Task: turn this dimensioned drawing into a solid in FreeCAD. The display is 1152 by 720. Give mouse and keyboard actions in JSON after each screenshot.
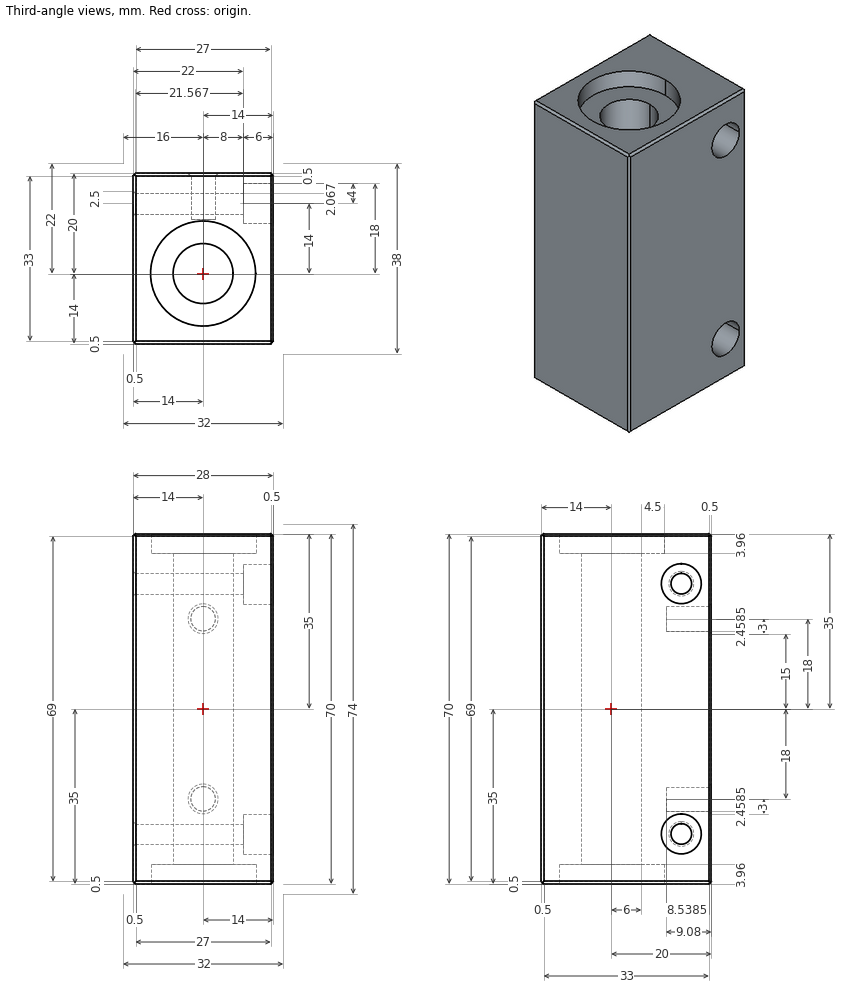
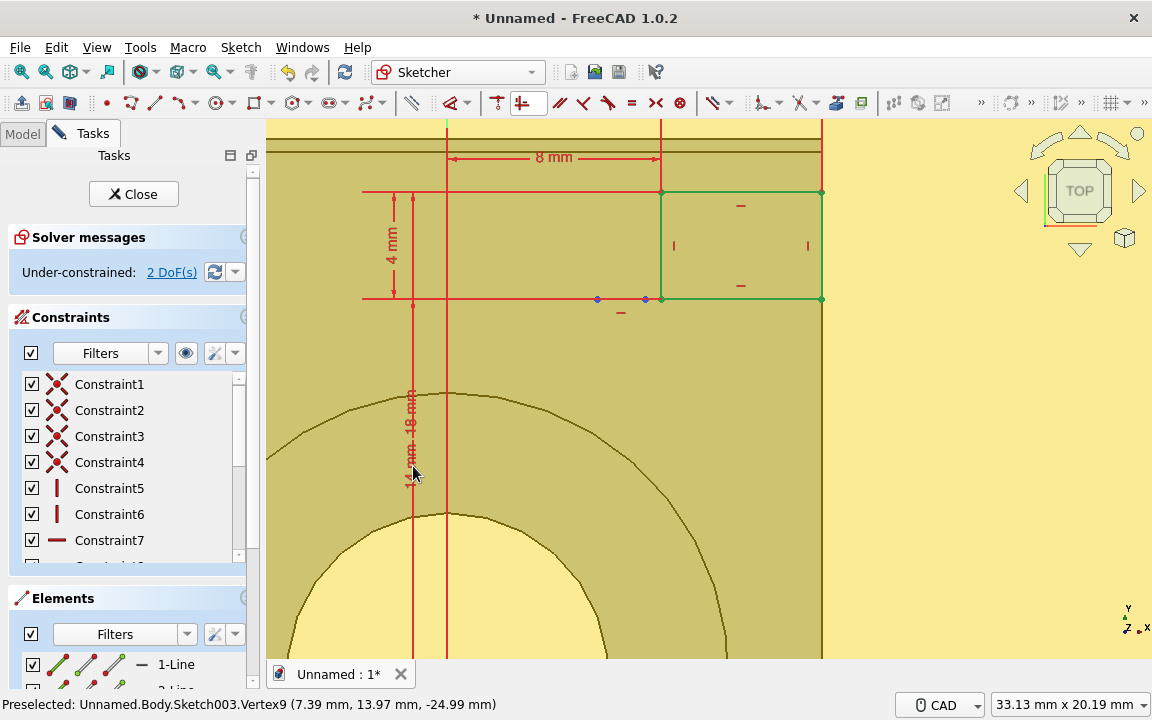
{"action": "left_click", "coordinate": [134, 194]}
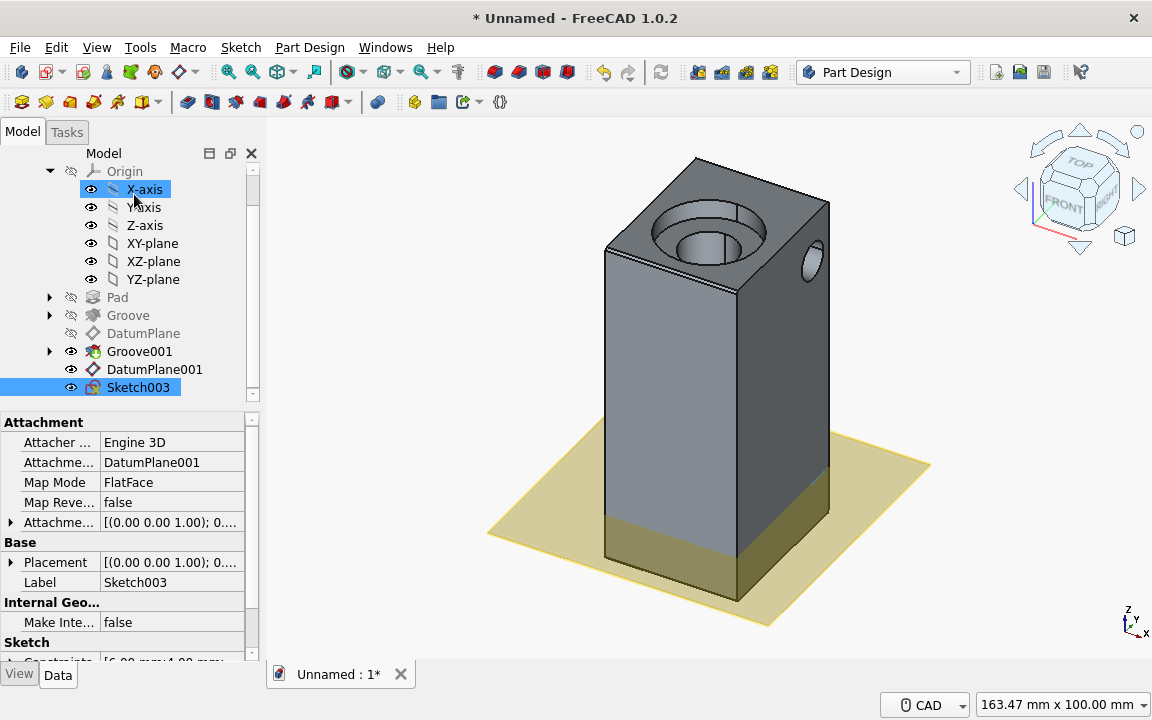
{"action": "left_click", "coordinate": [236, 102]}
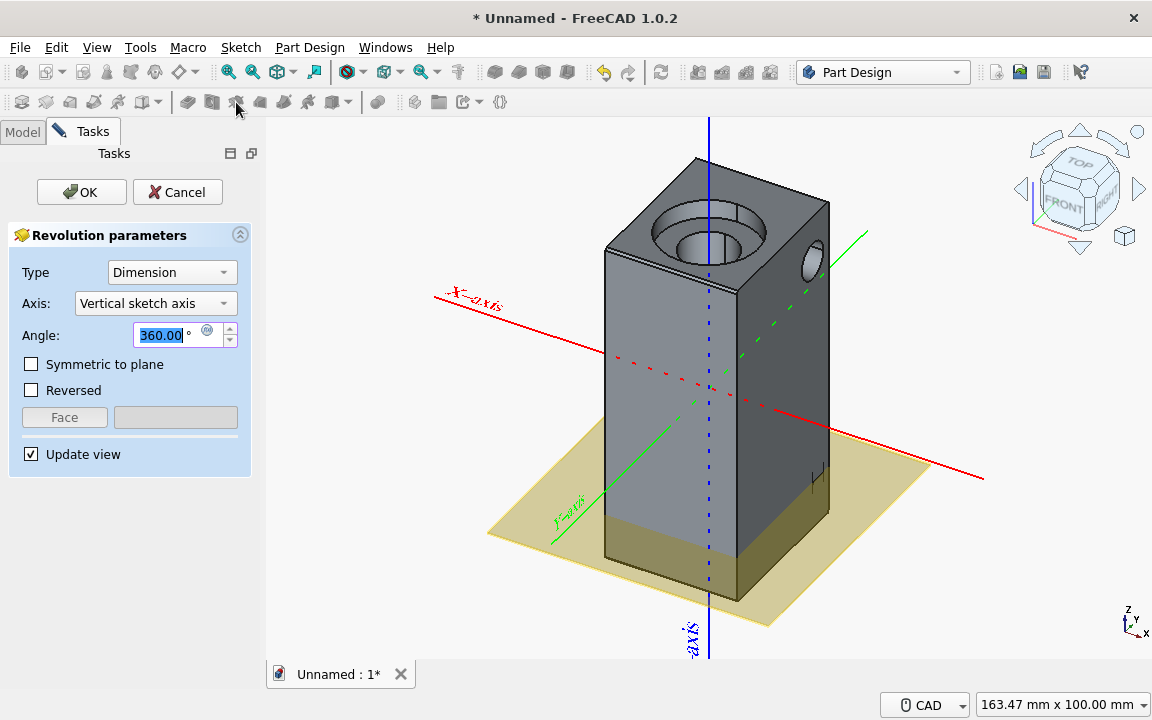
{"action": "left_click", "coordinate": [156, 304]}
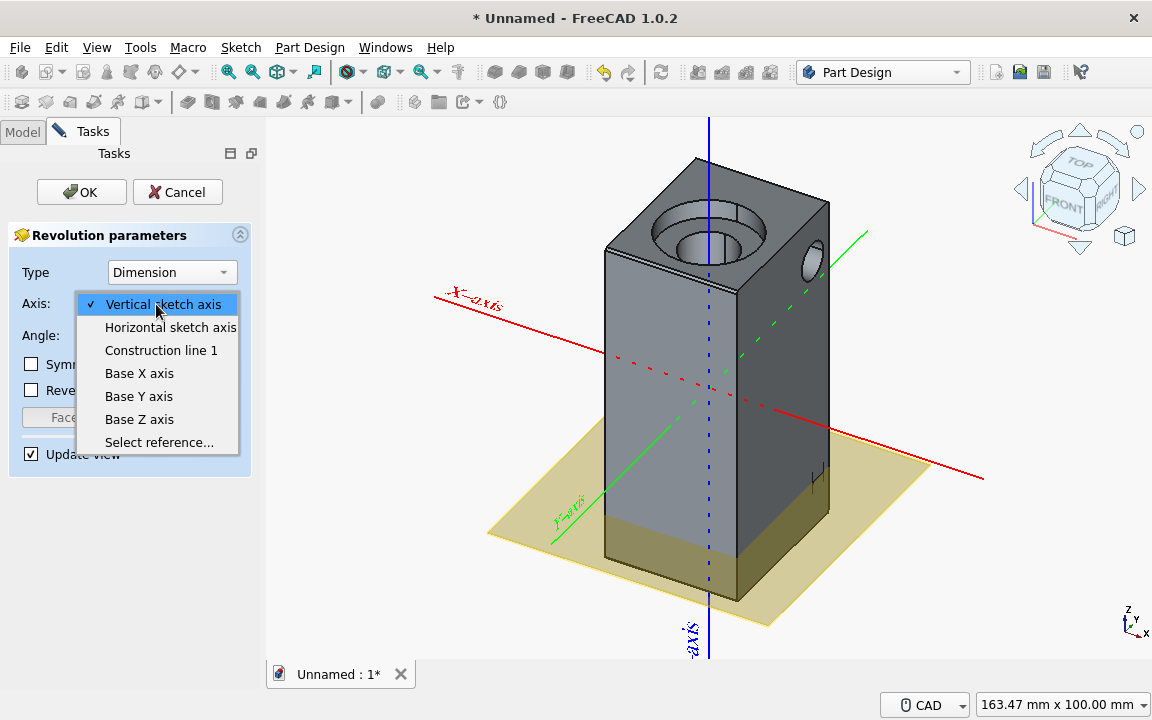
{"action": "left_click", "coordinate": [156, 350]}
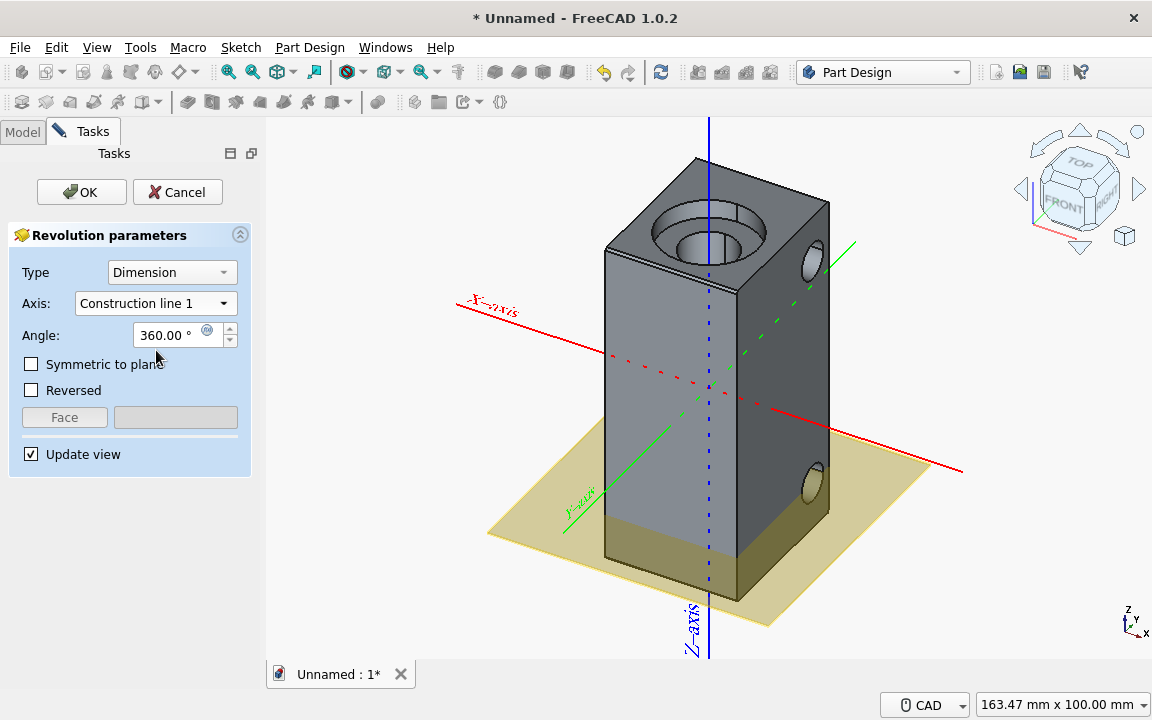
{"action": "left_click", "coordinate": [82, 192]}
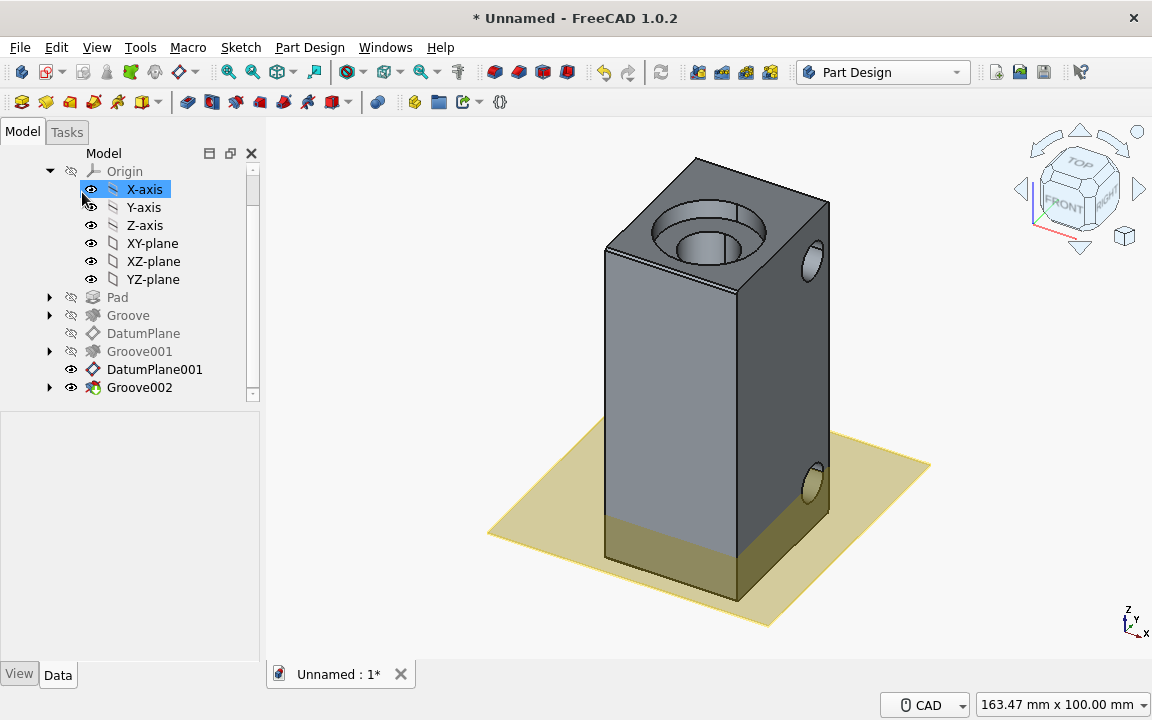
{"action": "left_click", "coordinate": [116, 369]}
{"action": "key", "text": "space"}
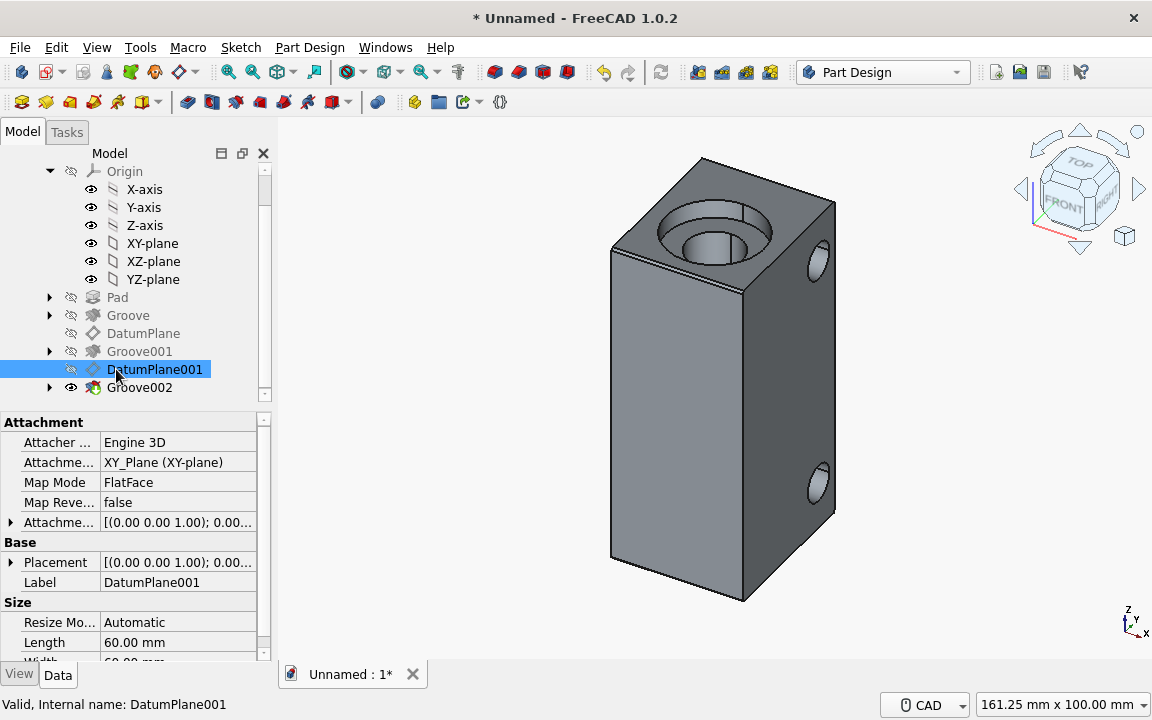
{"action": "left_click", "coordinate": [318, 619]}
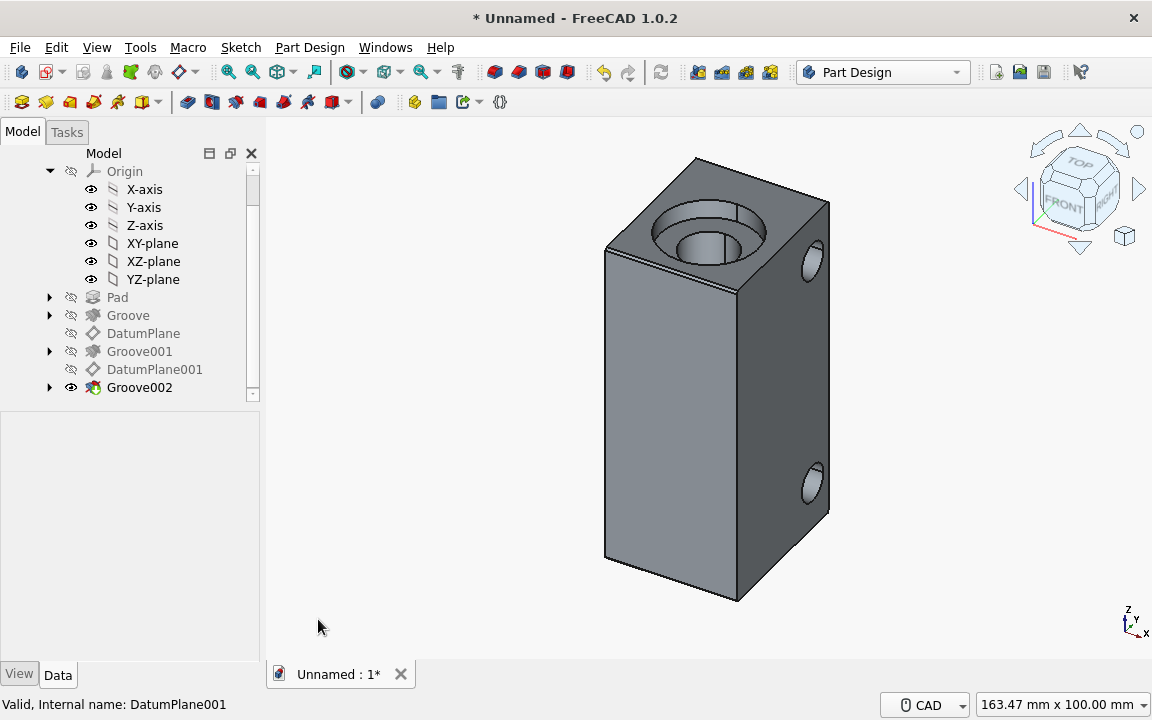
{"action": "left_click", "coordinate": [46, 72]}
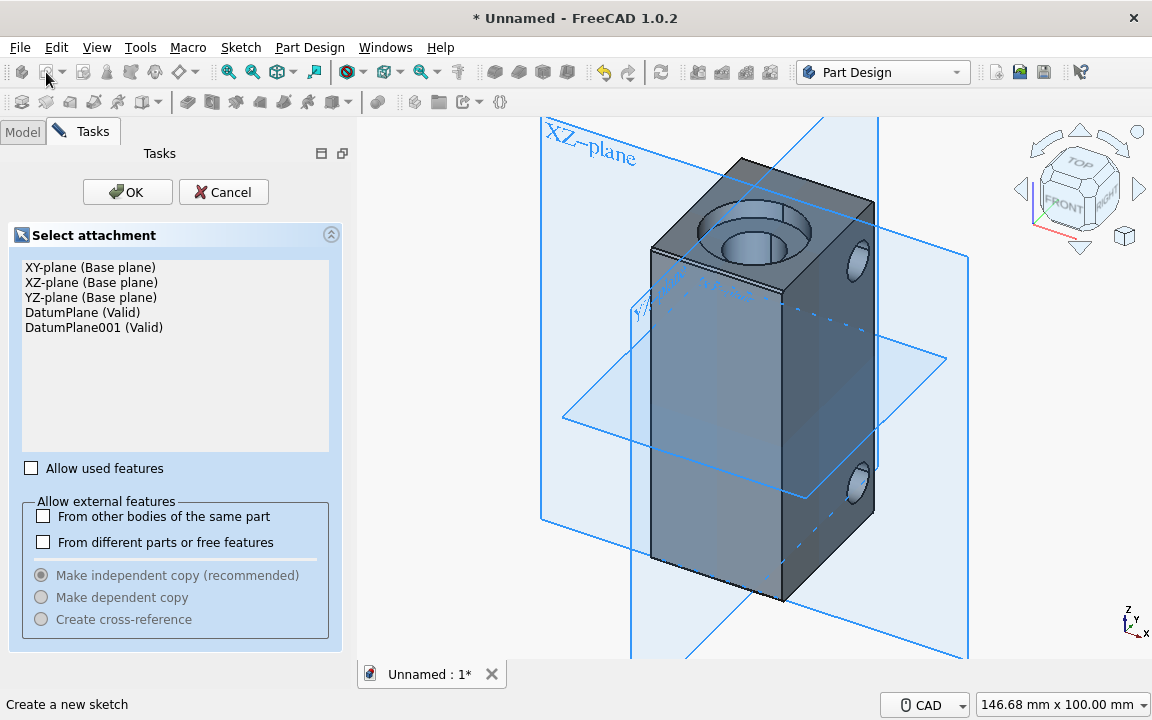
{"action": "left_click", "coordinate": [82, 298]}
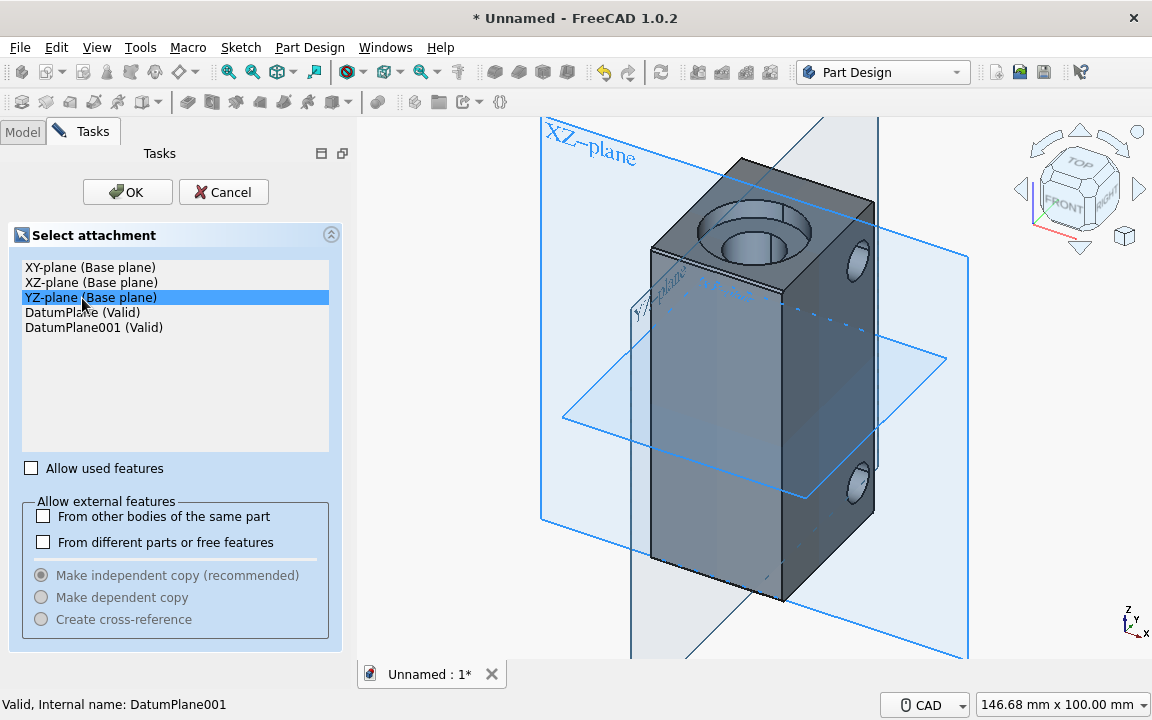
{"action": "left_click", "coordinate": [128, 192]}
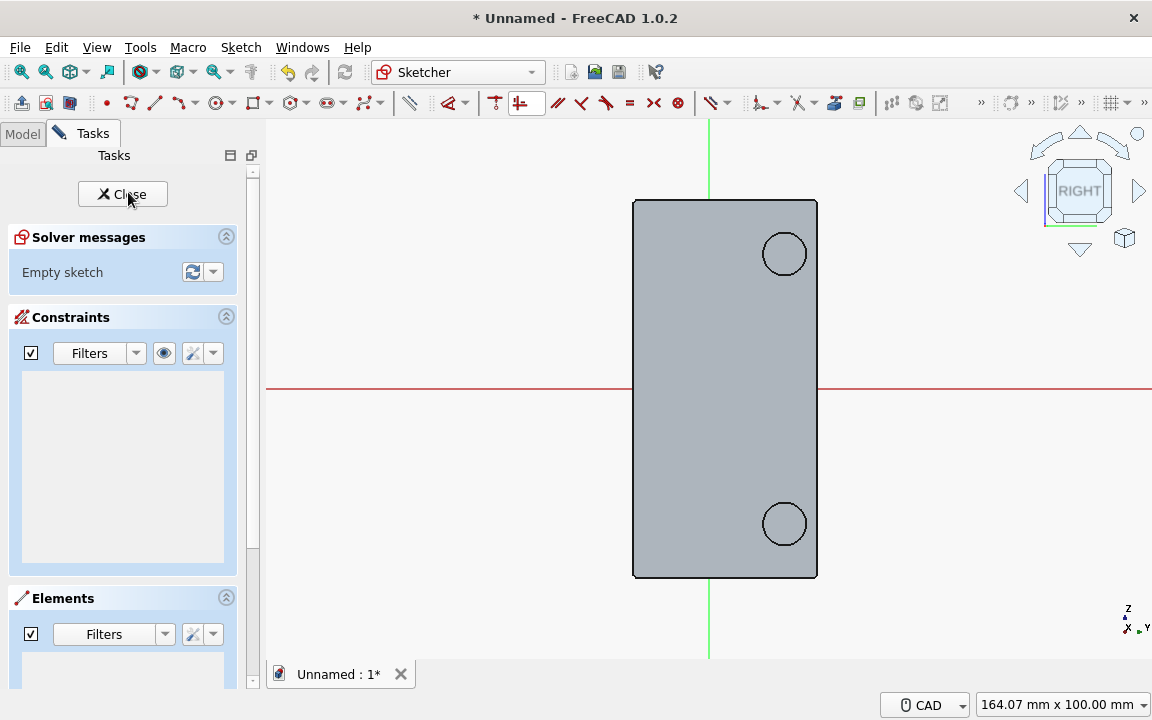
{"action": "left_click", "coordinate": [70, 104]}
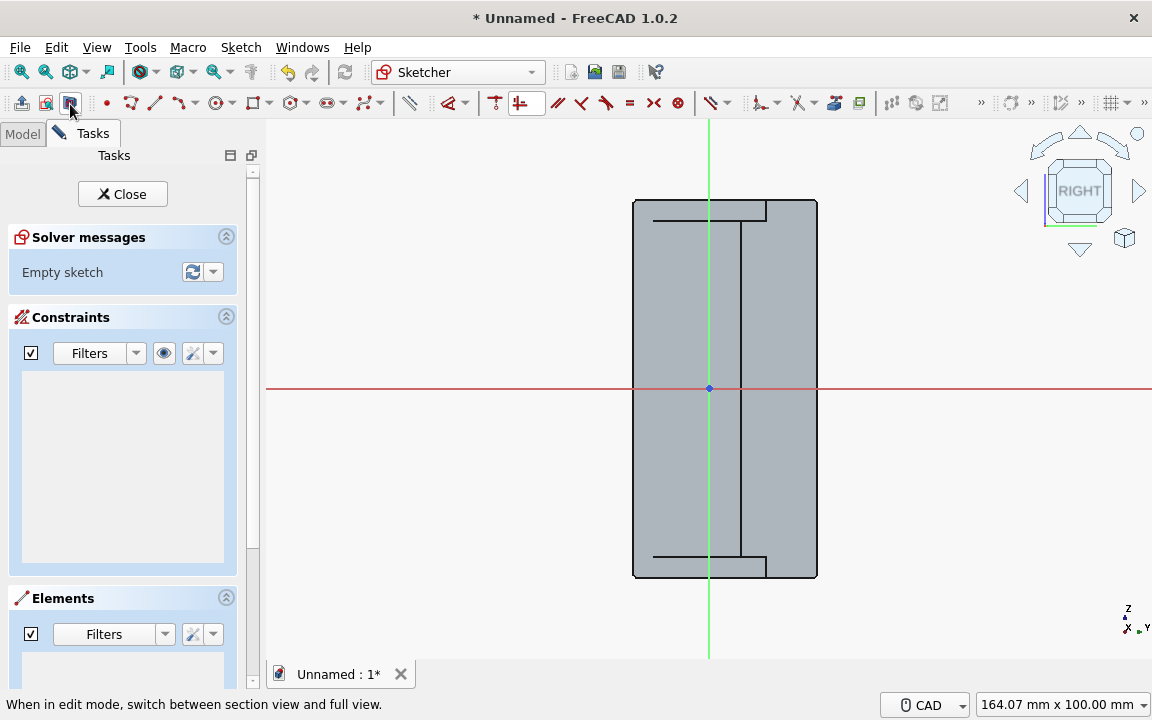
{"action": "scroll", "coordinate": [830, 470], "scroll_direction": "up", "scroll_amount": 6}